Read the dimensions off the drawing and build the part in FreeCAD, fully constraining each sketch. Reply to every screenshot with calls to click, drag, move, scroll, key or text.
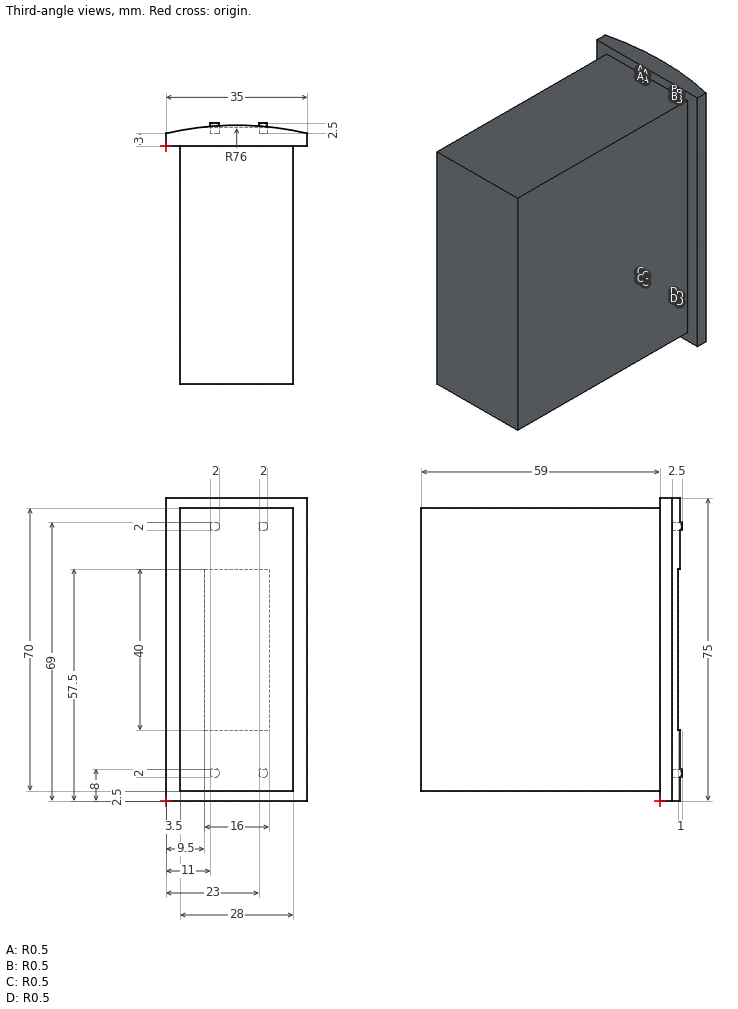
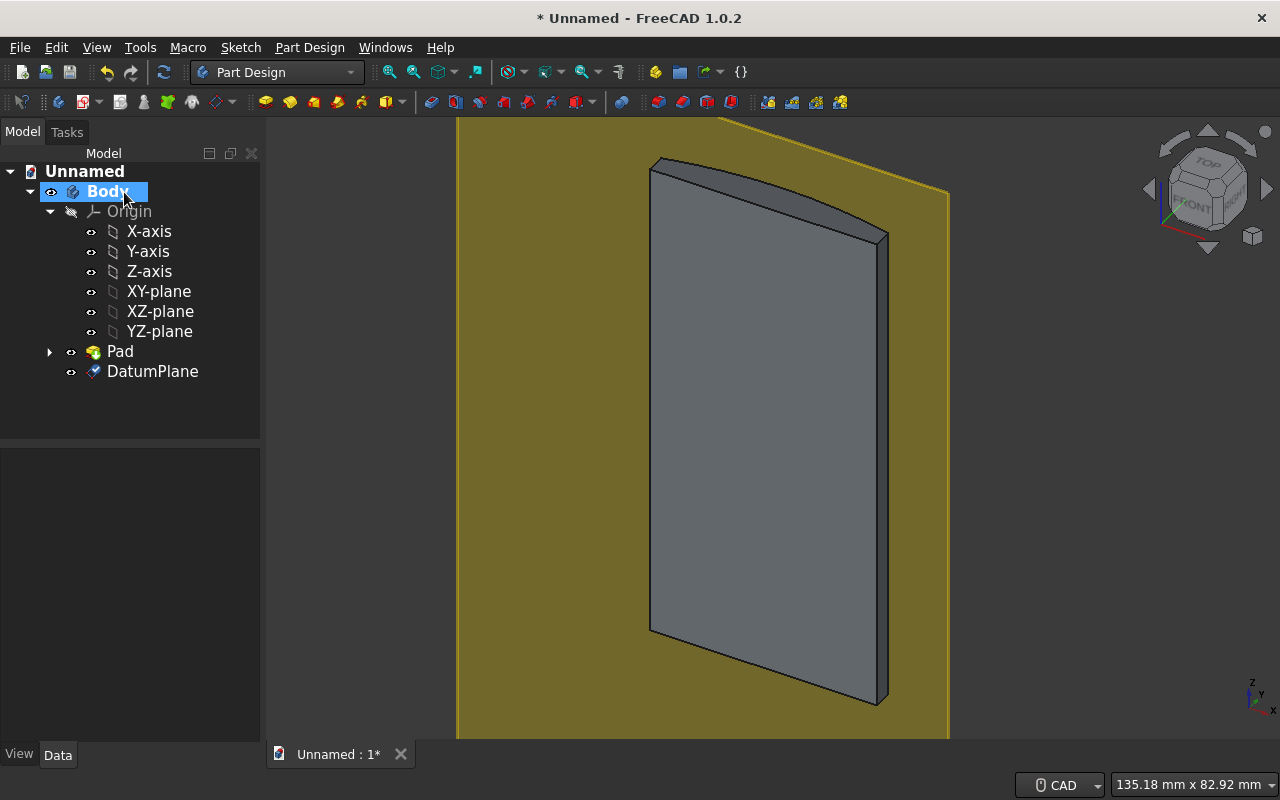
click(116, 372)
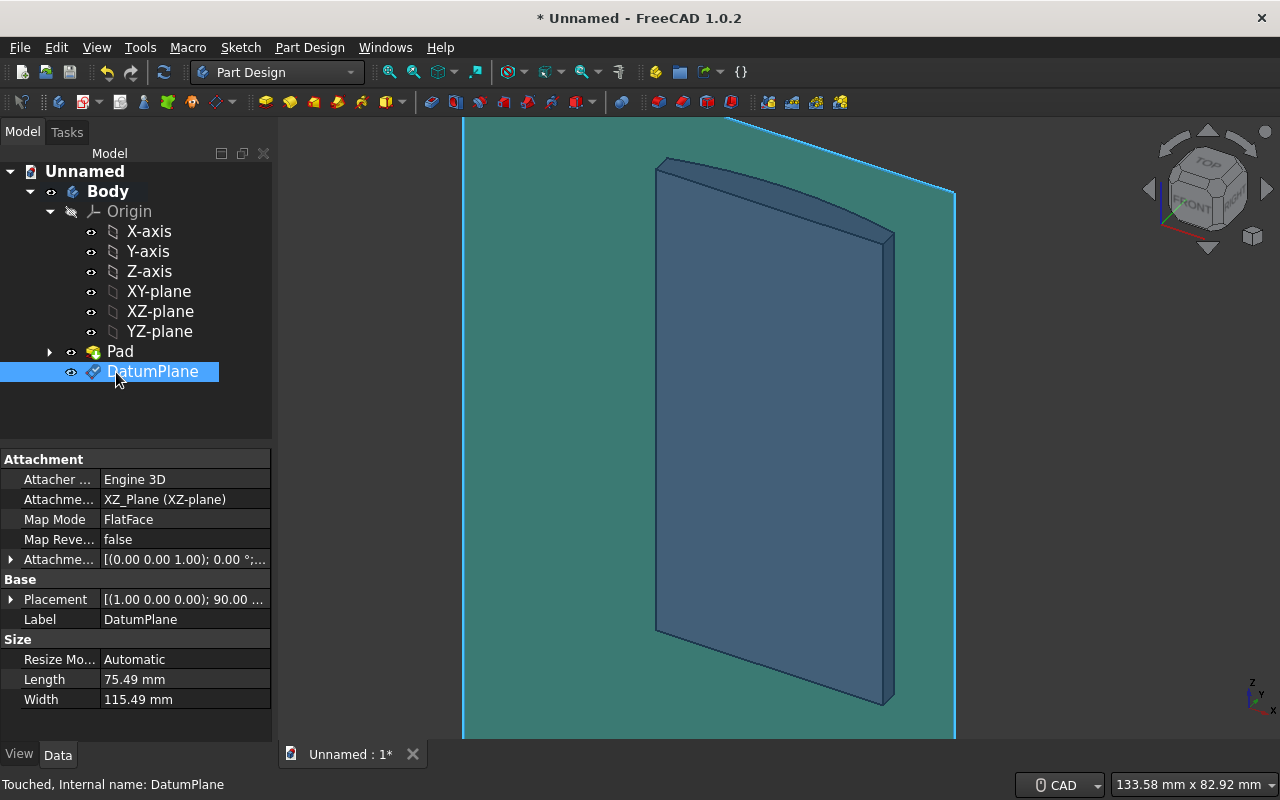
click(84, 102)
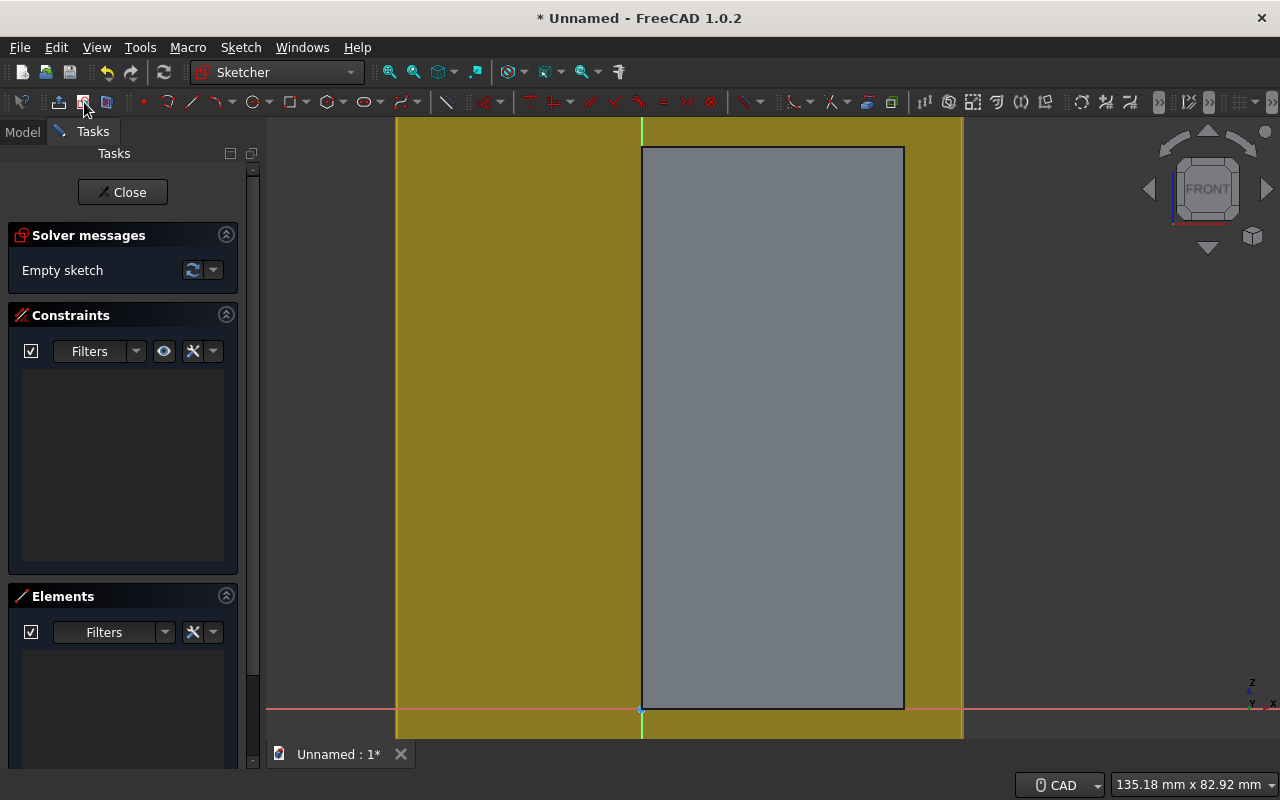
key(q)
key(s)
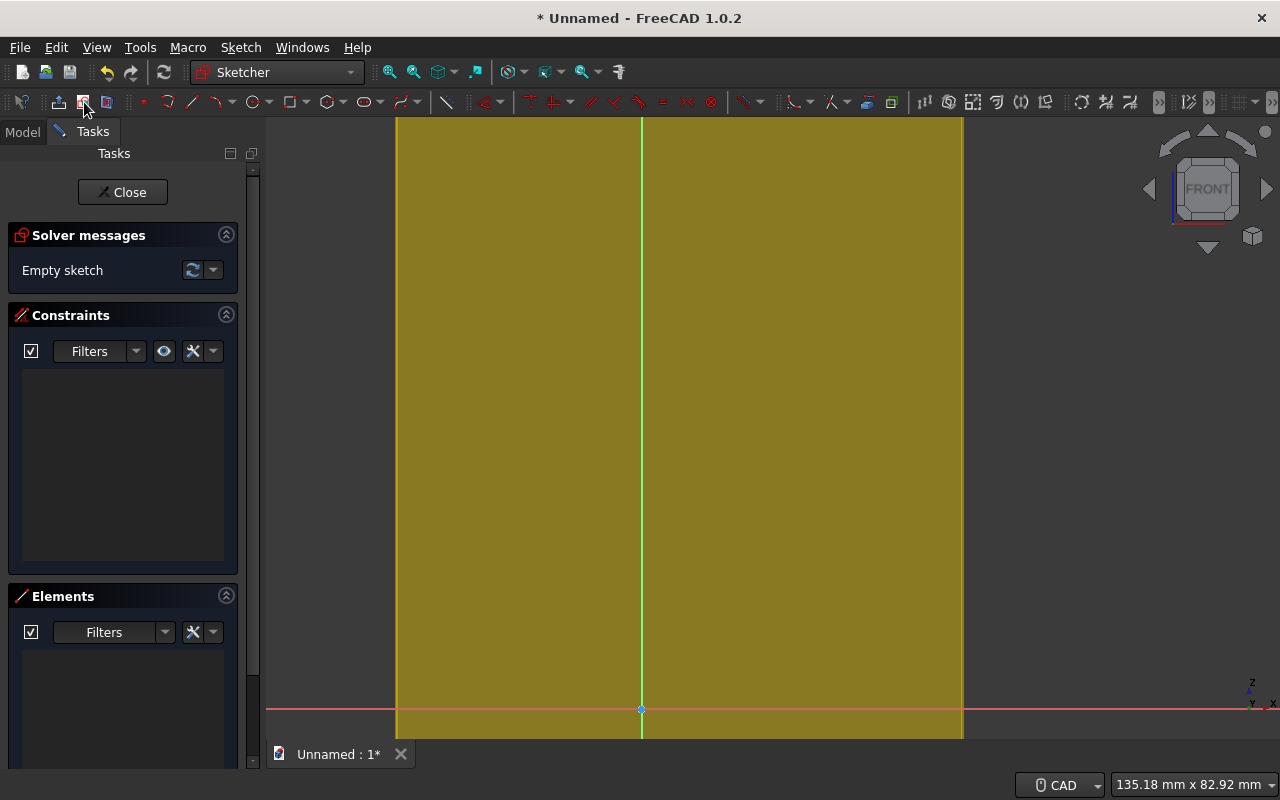
scroll(556, 145, down, 1)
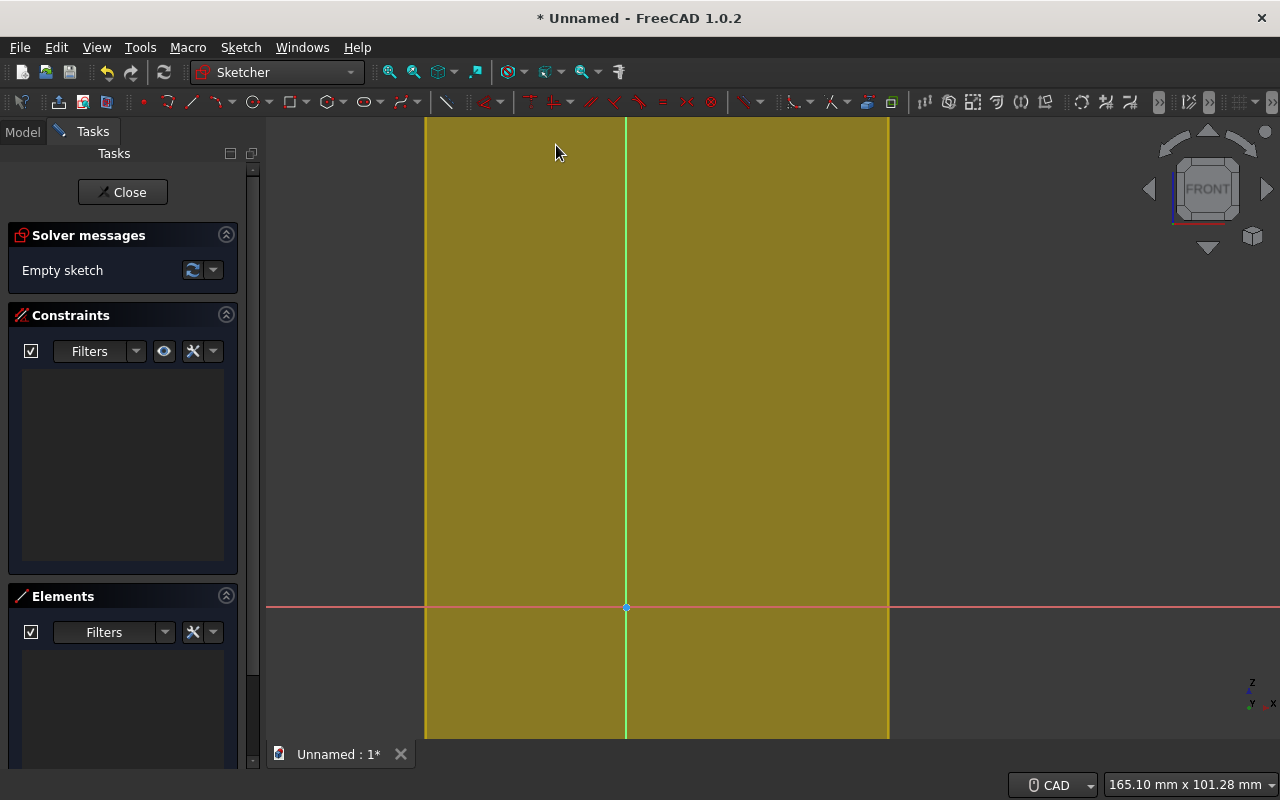
key(g)
key(r)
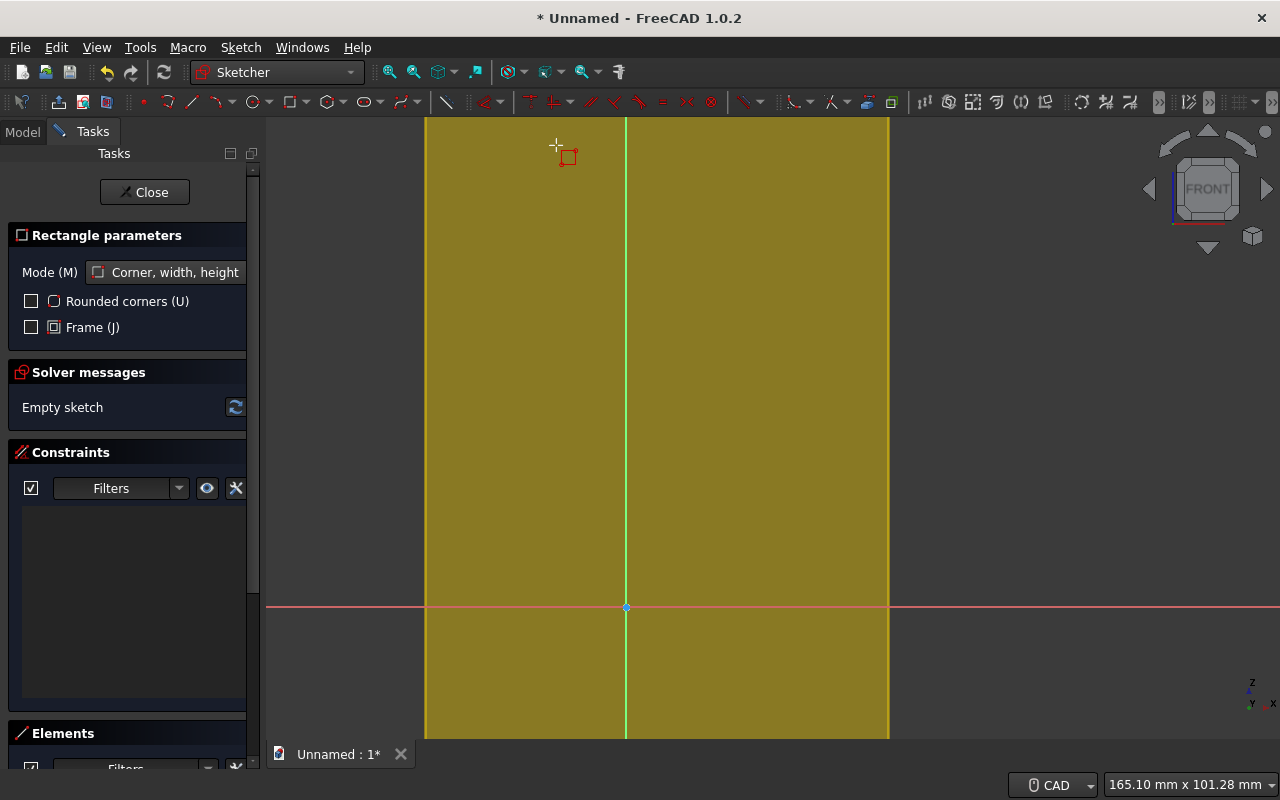
click(685, 254)
click(783, 500)
key(Escape)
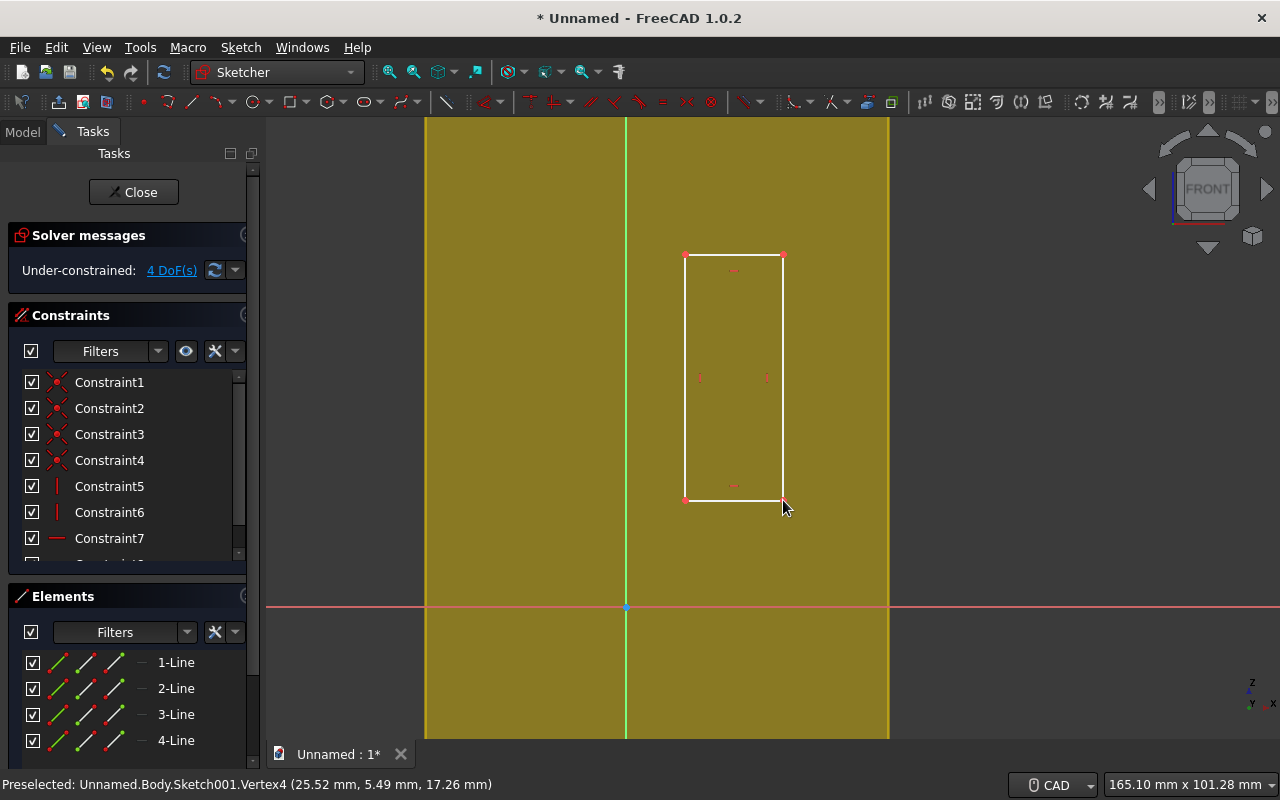
click(484, 102)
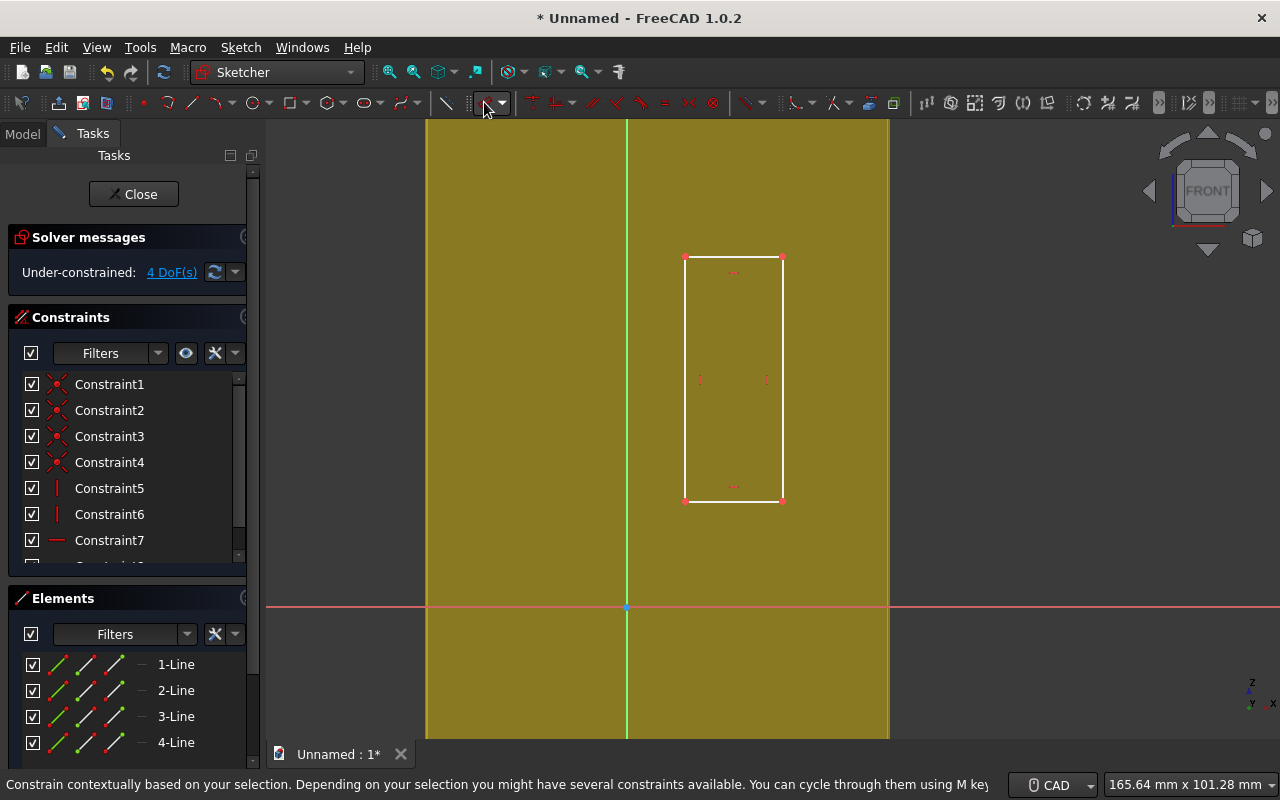
click(685, 330)
click(651, 379)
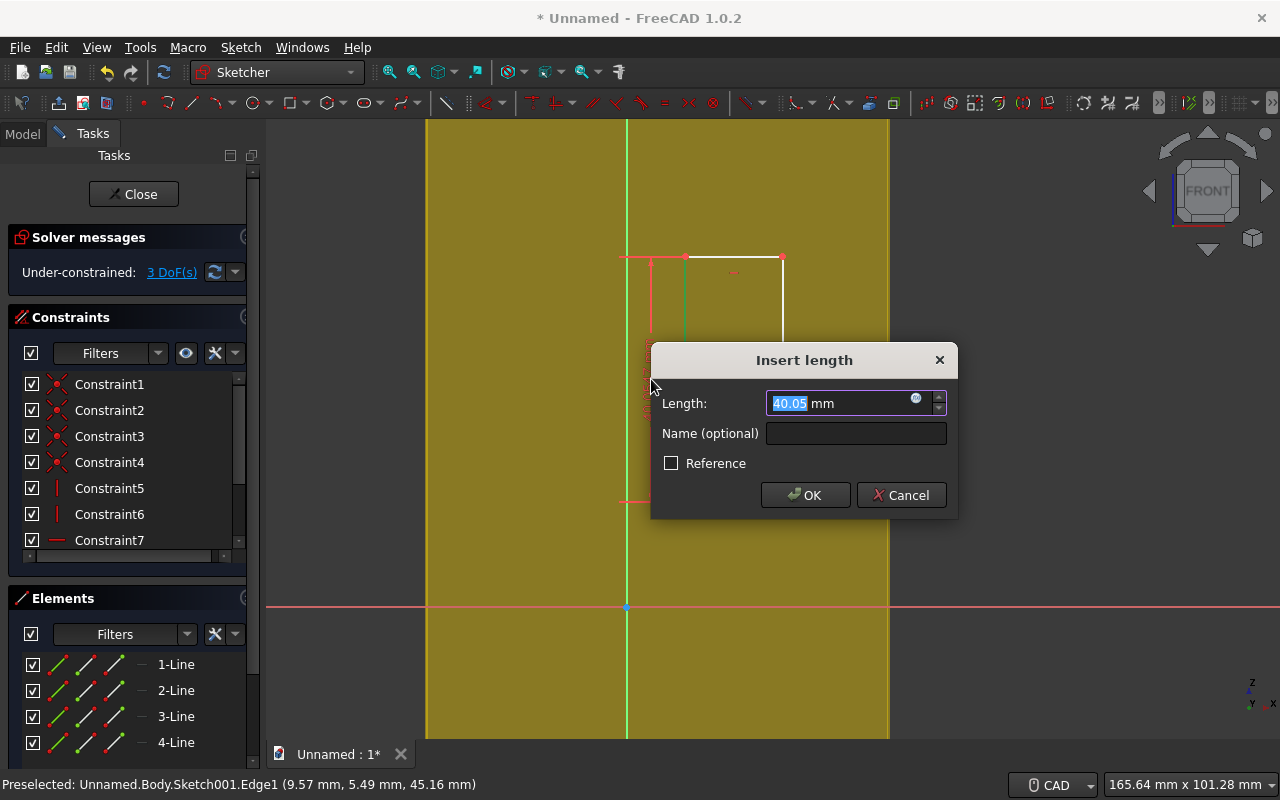
text(40)
key(Return)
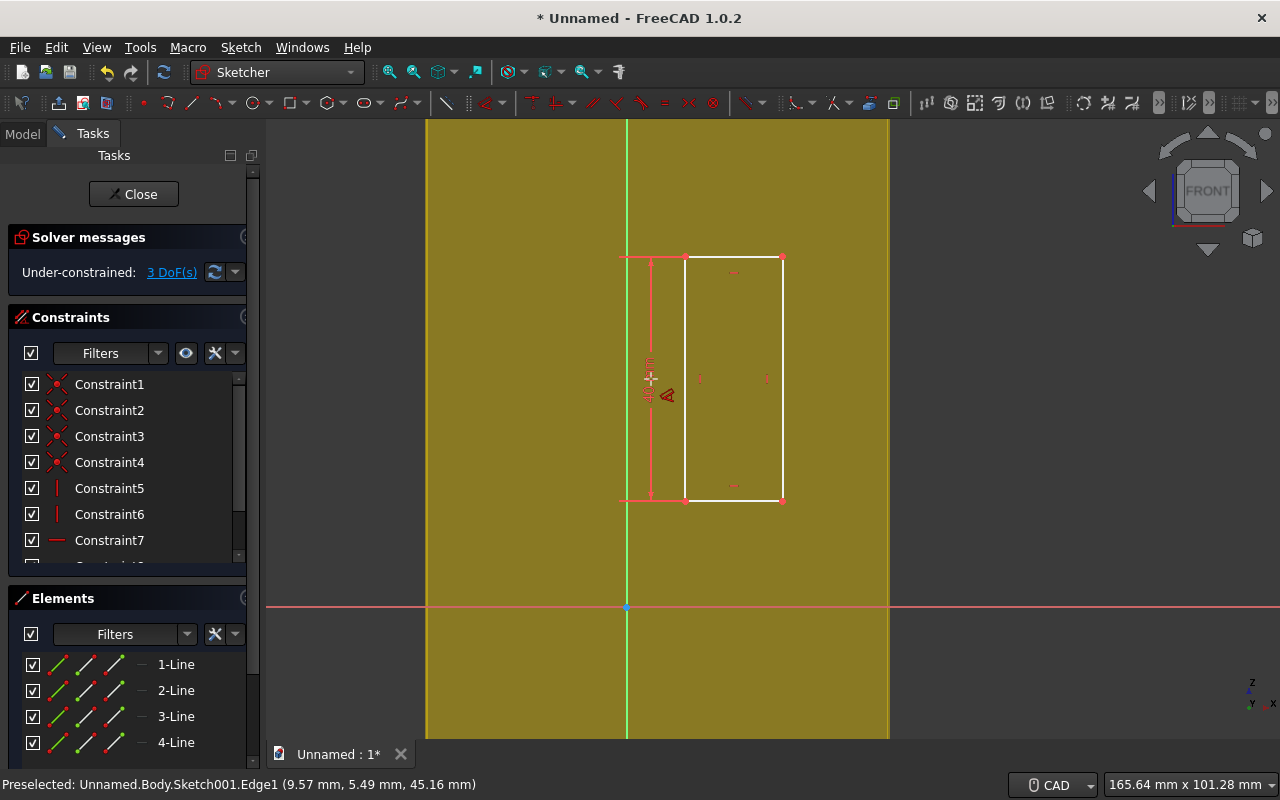
click(715, 501)
click(734, 535)